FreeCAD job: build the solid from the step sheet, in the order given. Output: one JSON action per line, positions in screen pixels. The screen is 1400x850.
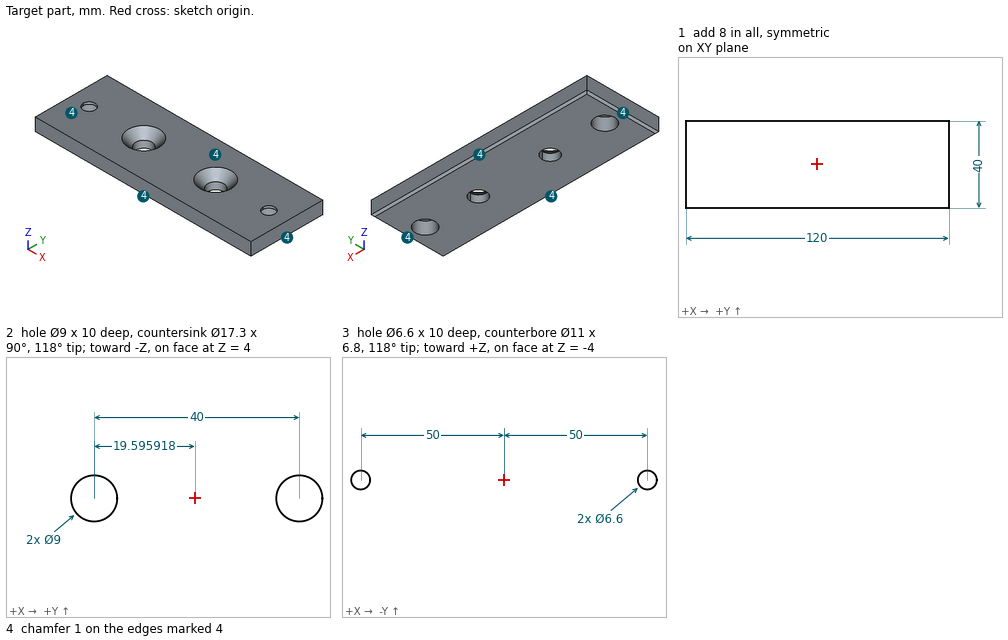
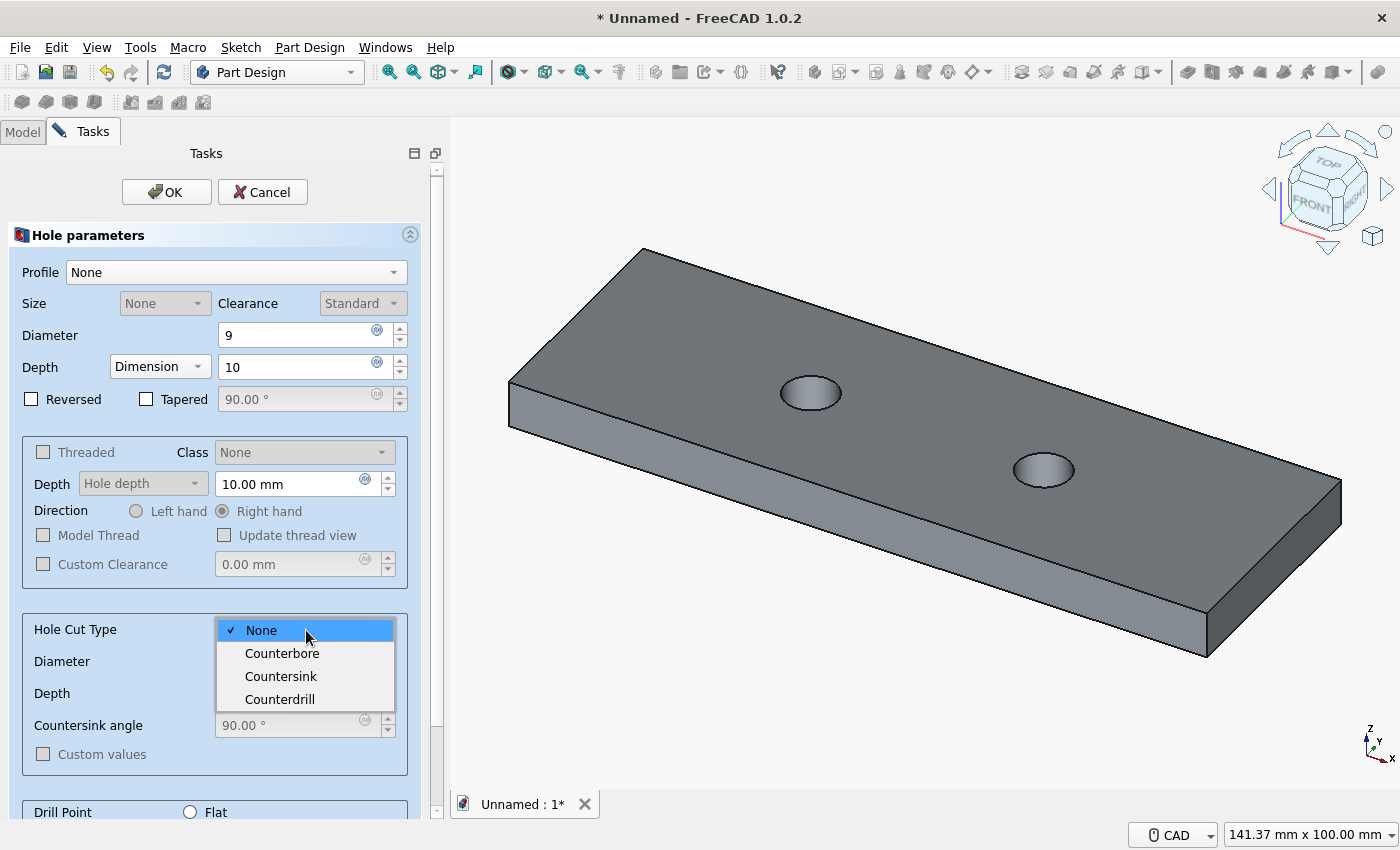
{"action": "left_click", "coordinate": [304, 676]}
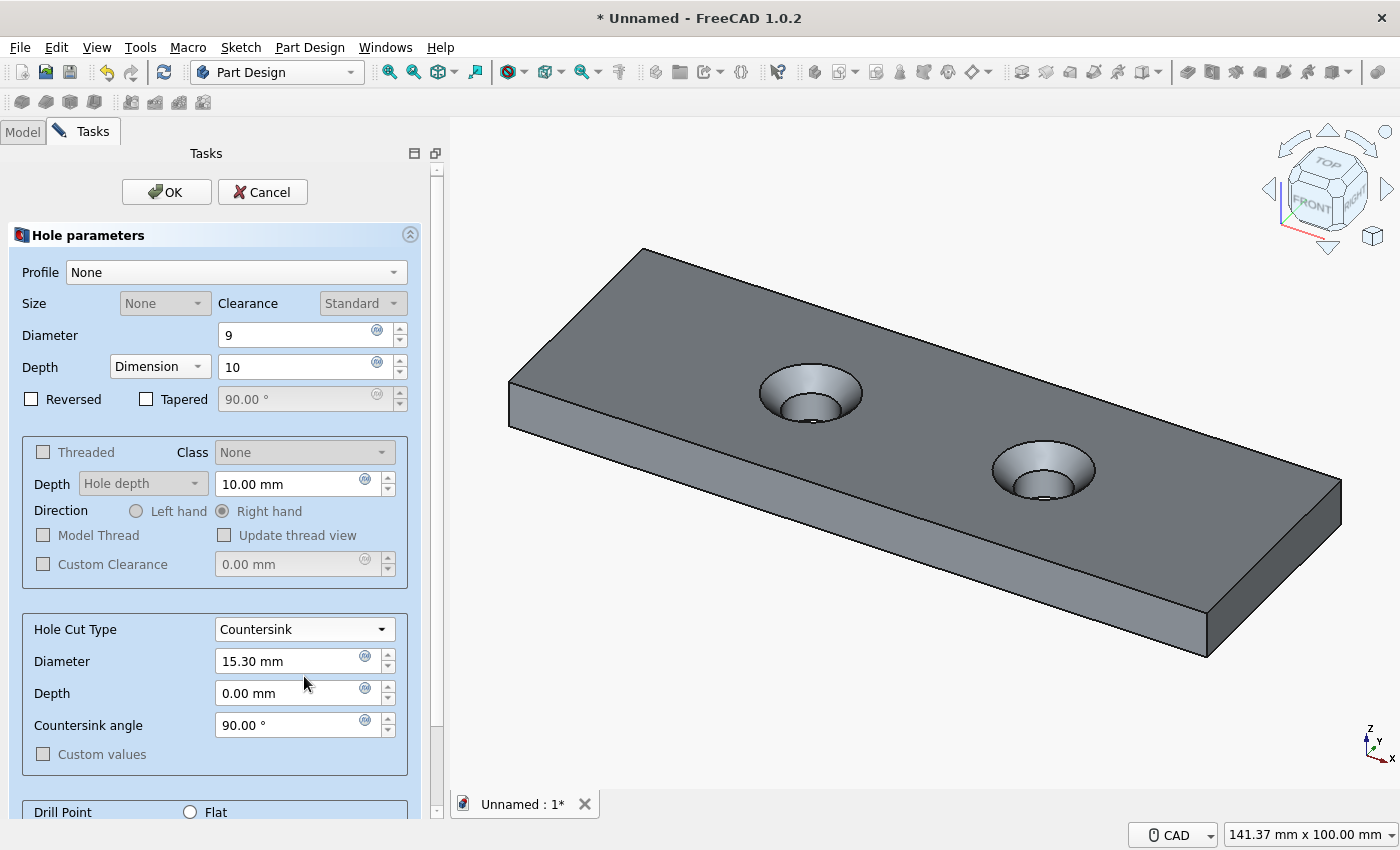
{"action": "triple_click", "coordinate": [298, 661]}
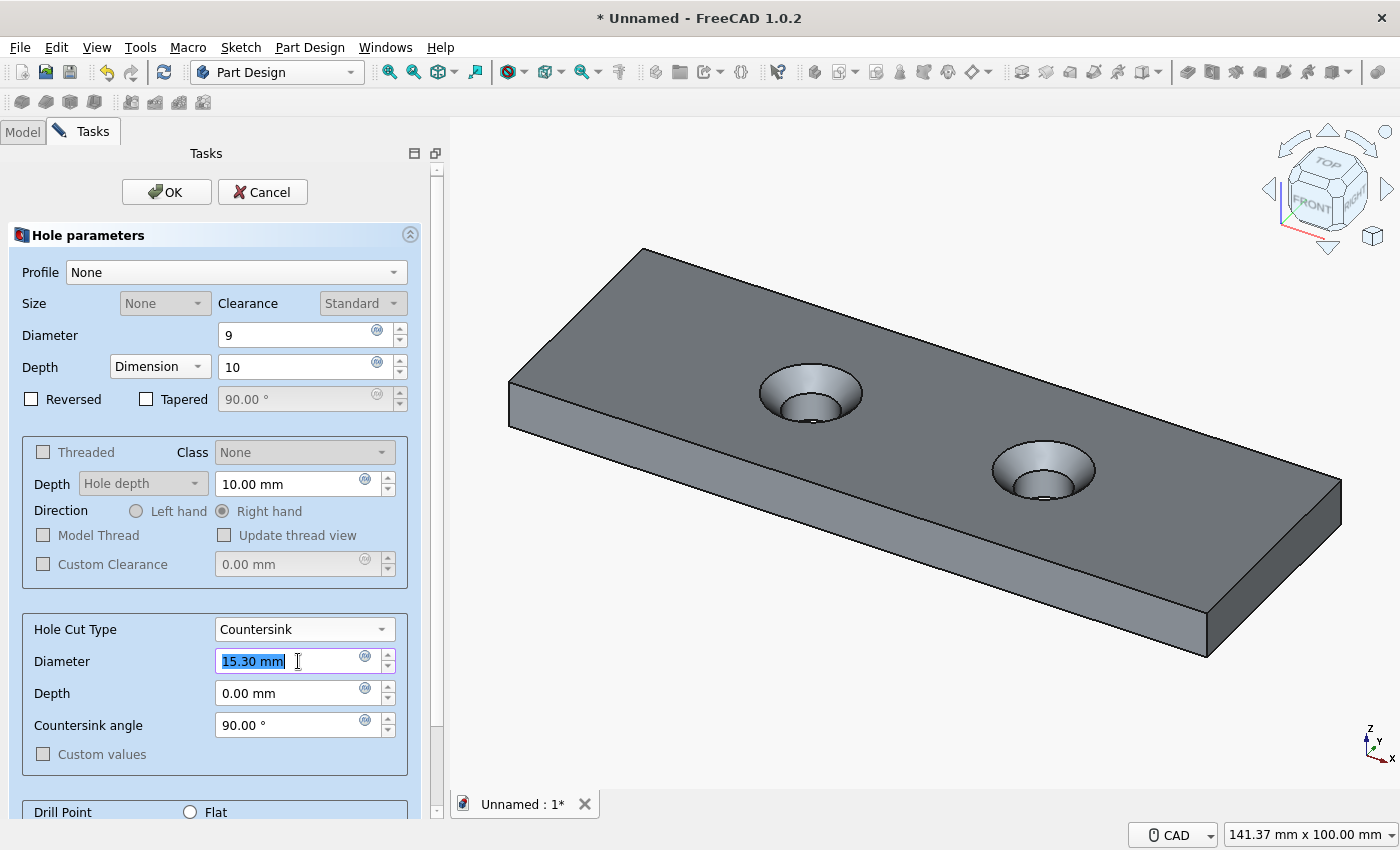
{"action": "type", "text": "17.3"}
{"action": "key", "text": "Tab"}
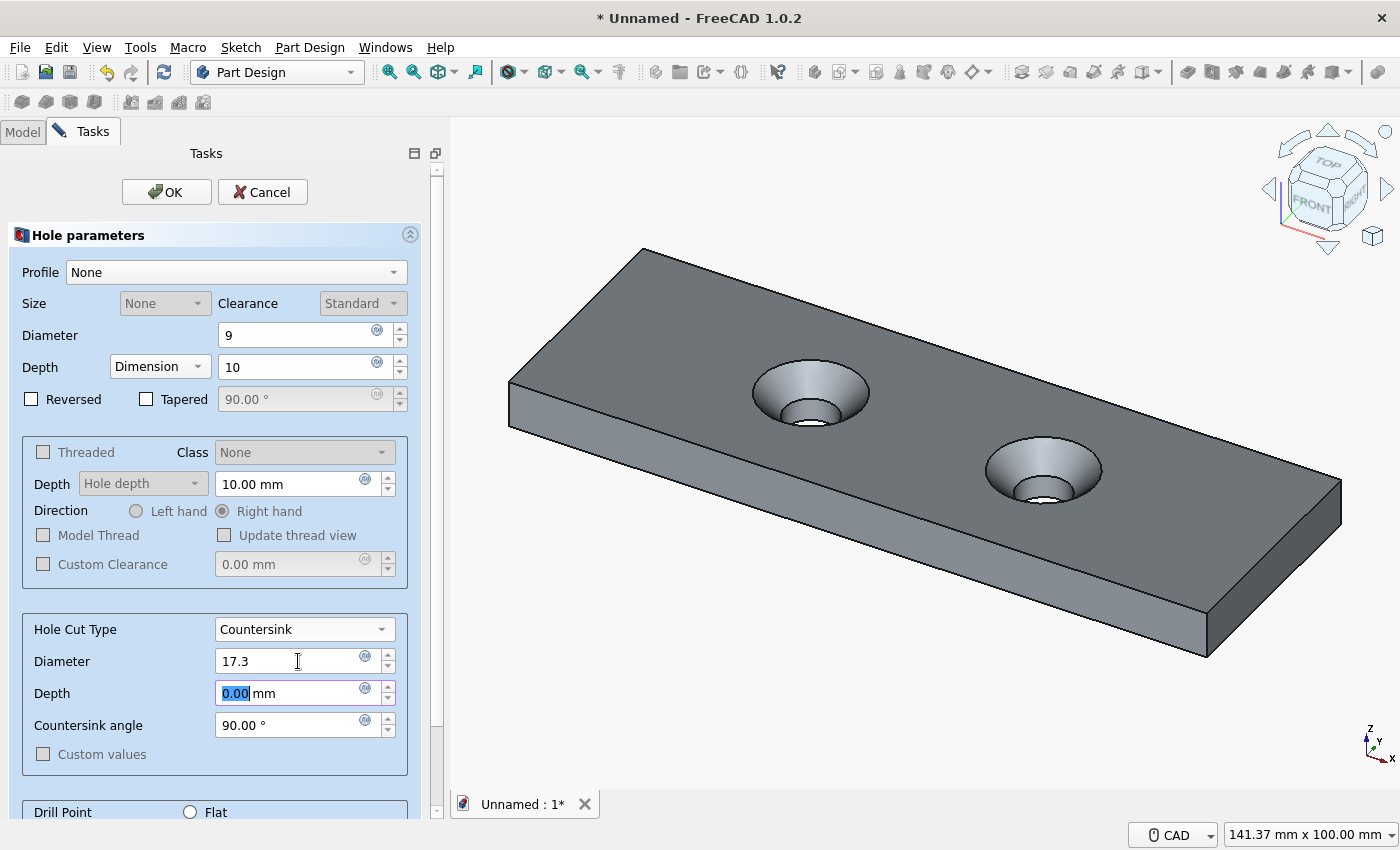
{"action": "left_click", "coordinate": [167, 192]}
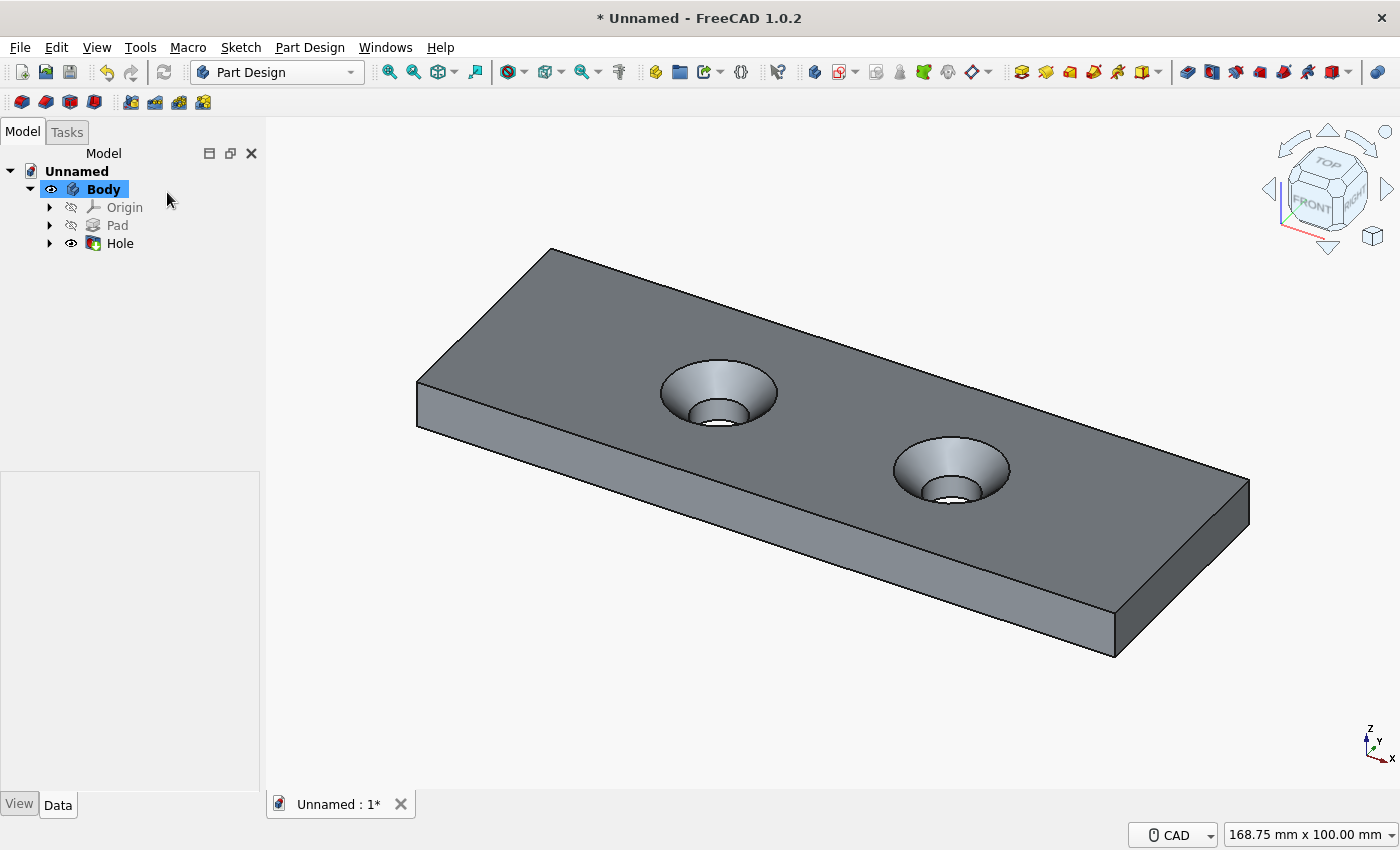
{"action": "key", "text": "5"}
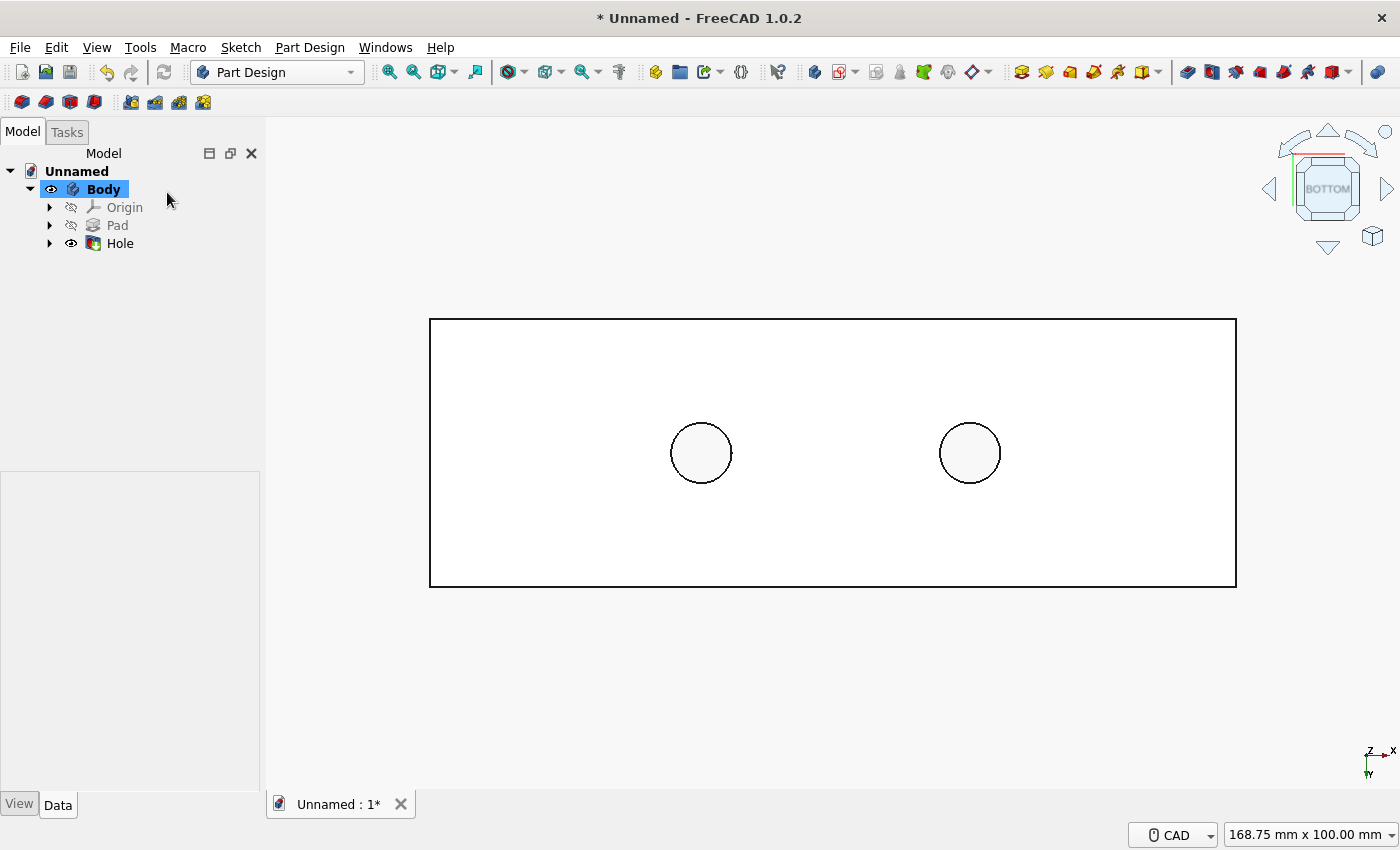
{"action": "left_click", "coordinate": [833, 452]}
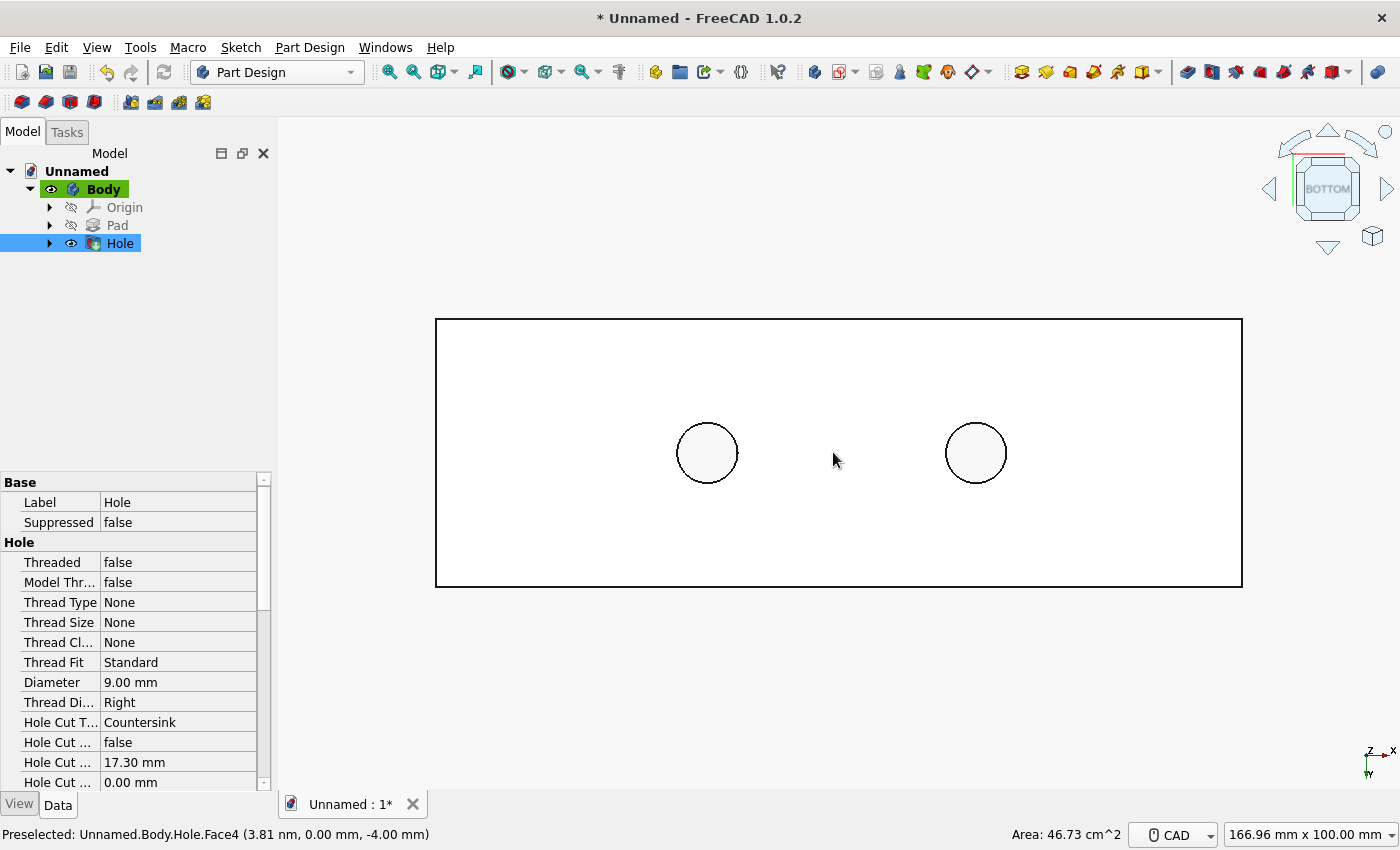
{"action": "left_click", "coordinate": [840, 72]}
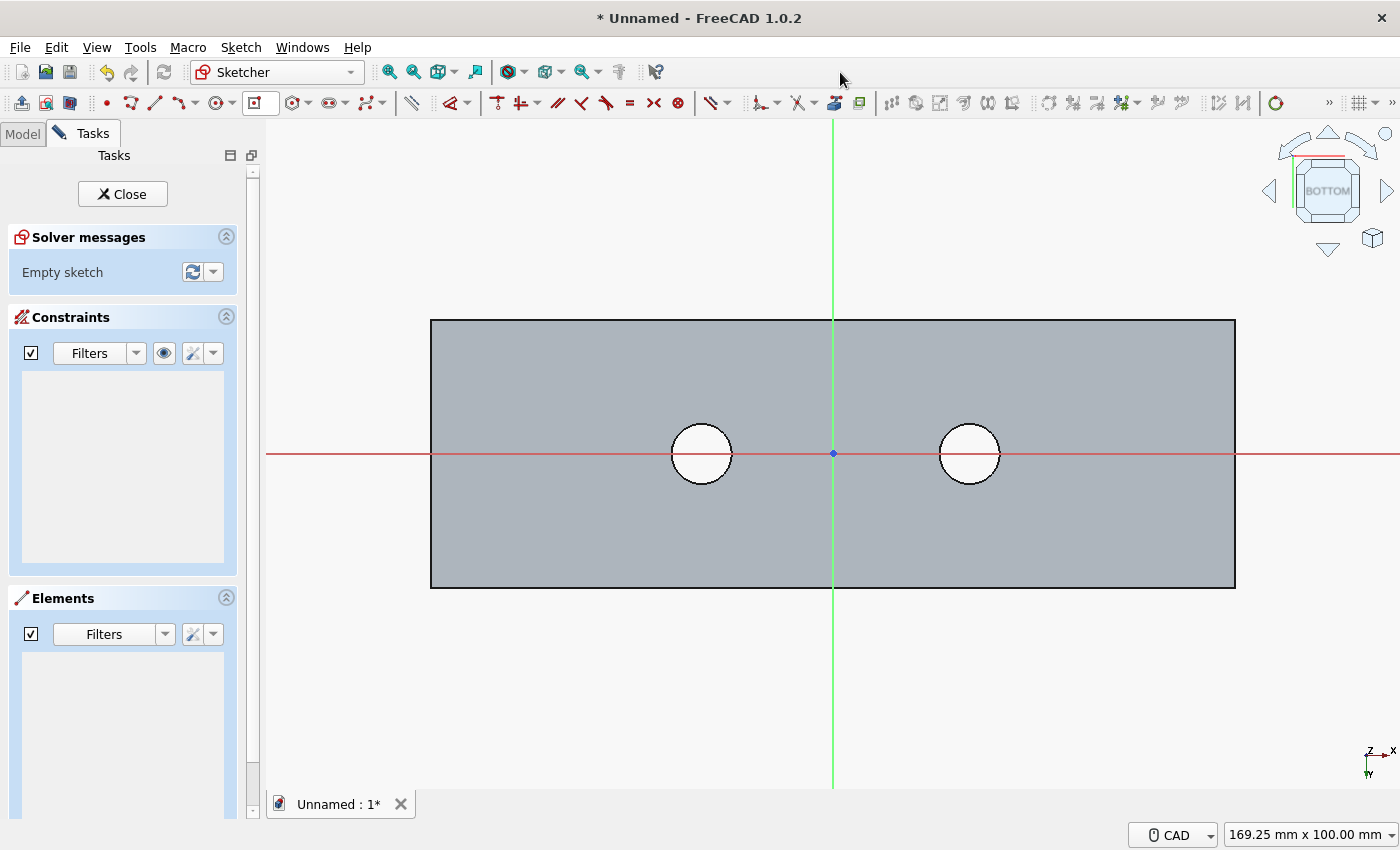
{"action": "left_click", "coordinate": [216, 104]}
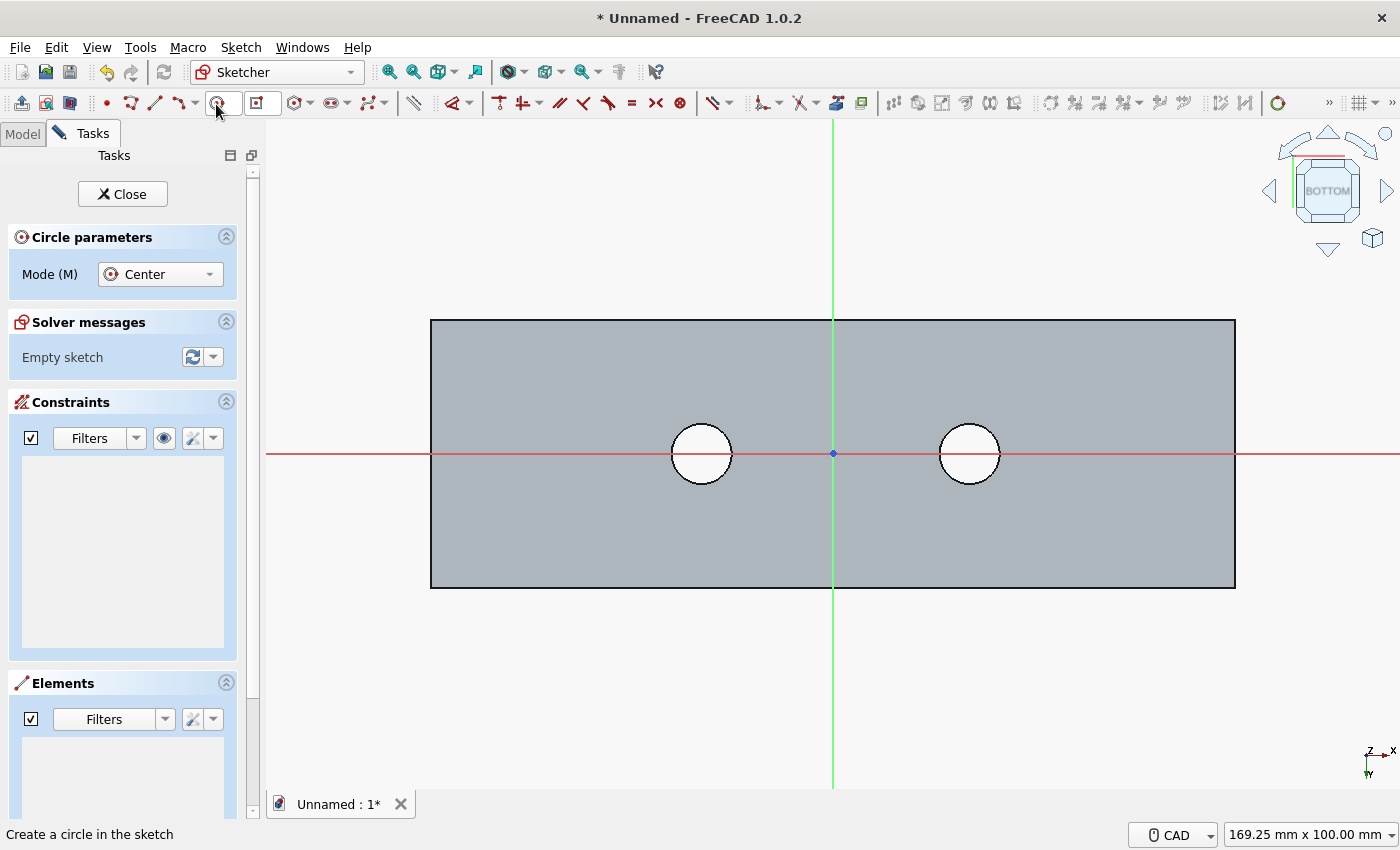
{"action": "left_click", "coordinate": [1168, 454]}
{"action": "left_click", "coordinate": [1184, 438]}